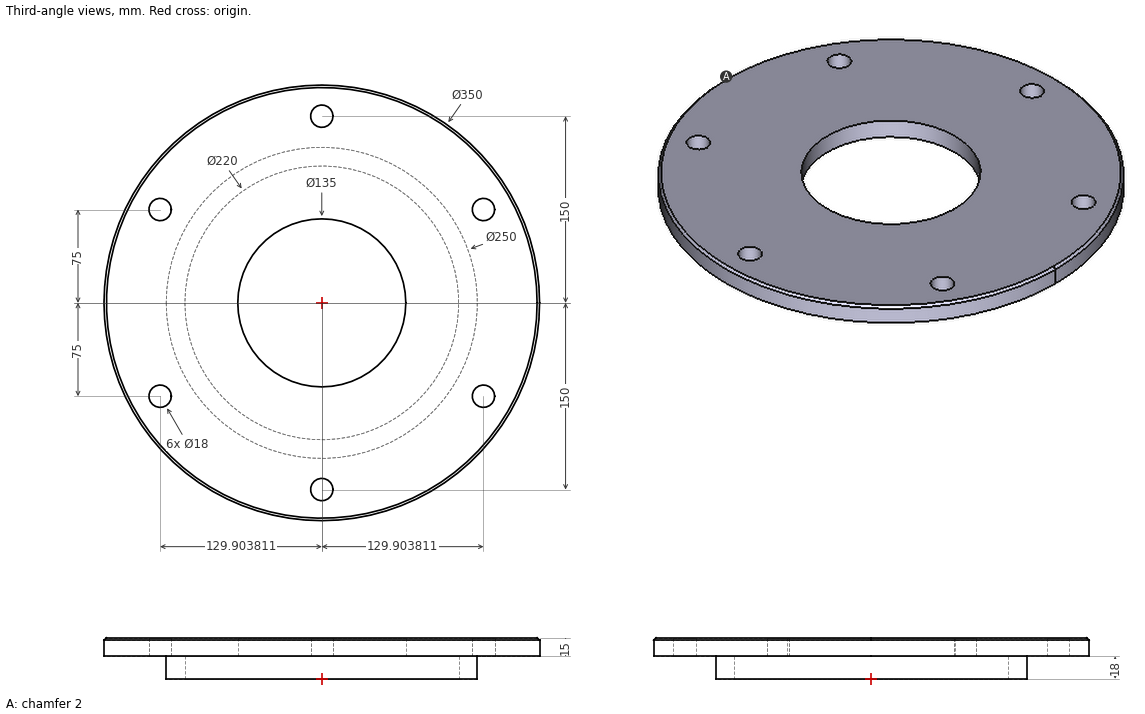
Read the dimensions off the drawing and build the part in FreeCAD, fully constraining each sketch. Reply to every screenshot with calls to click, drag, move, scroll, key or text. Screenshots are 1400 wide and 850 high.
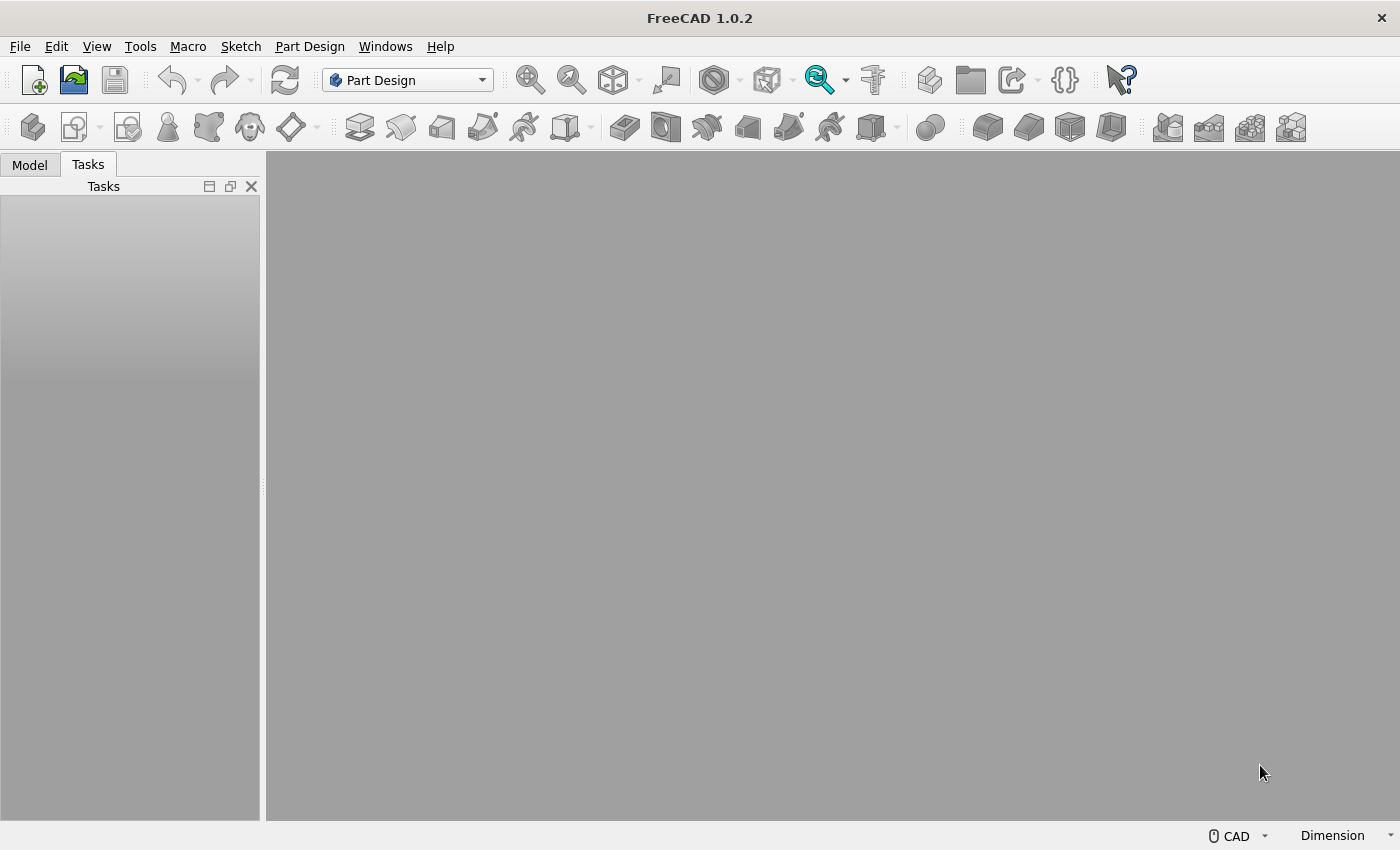
click(33, 80)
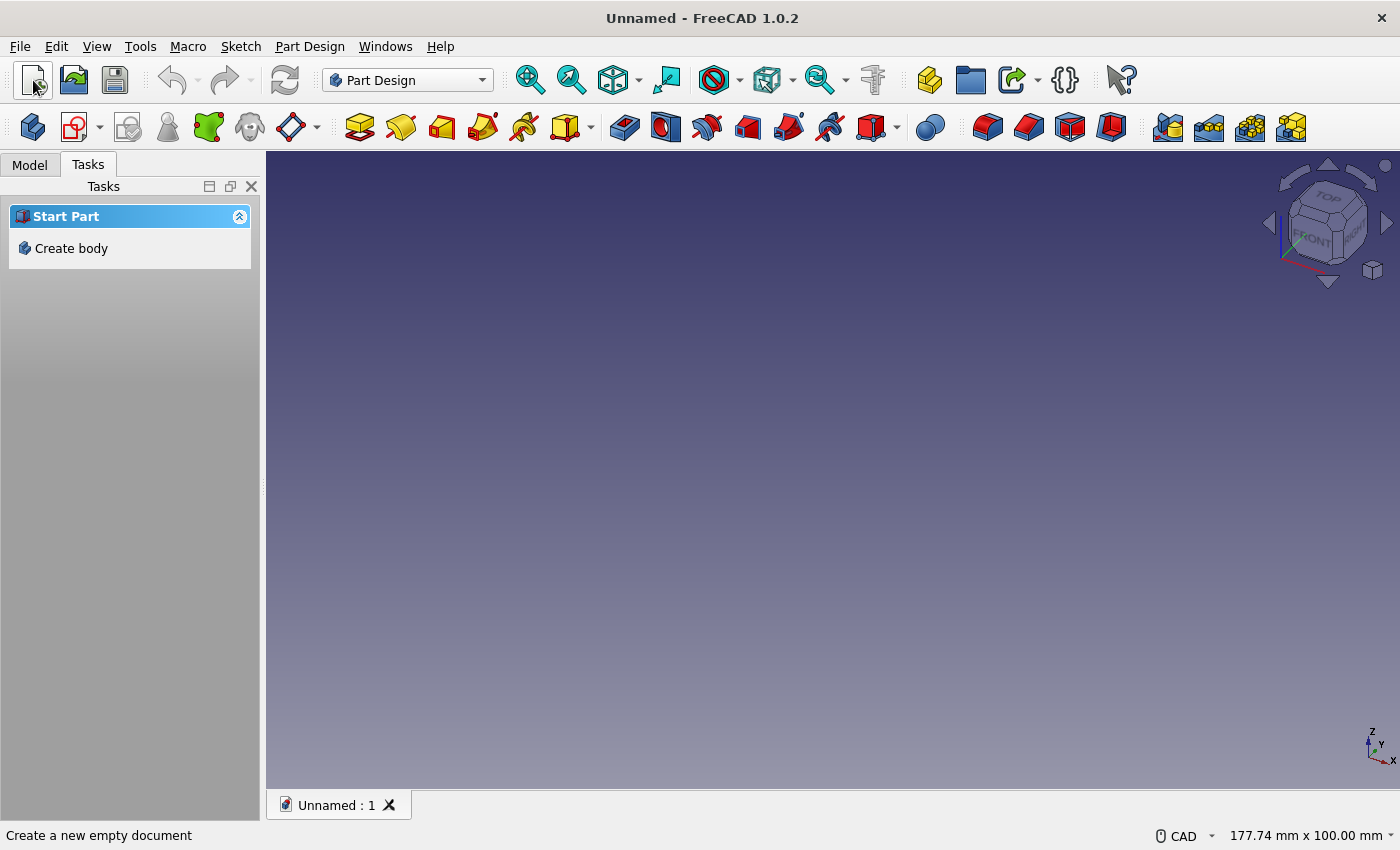
click(74, 128)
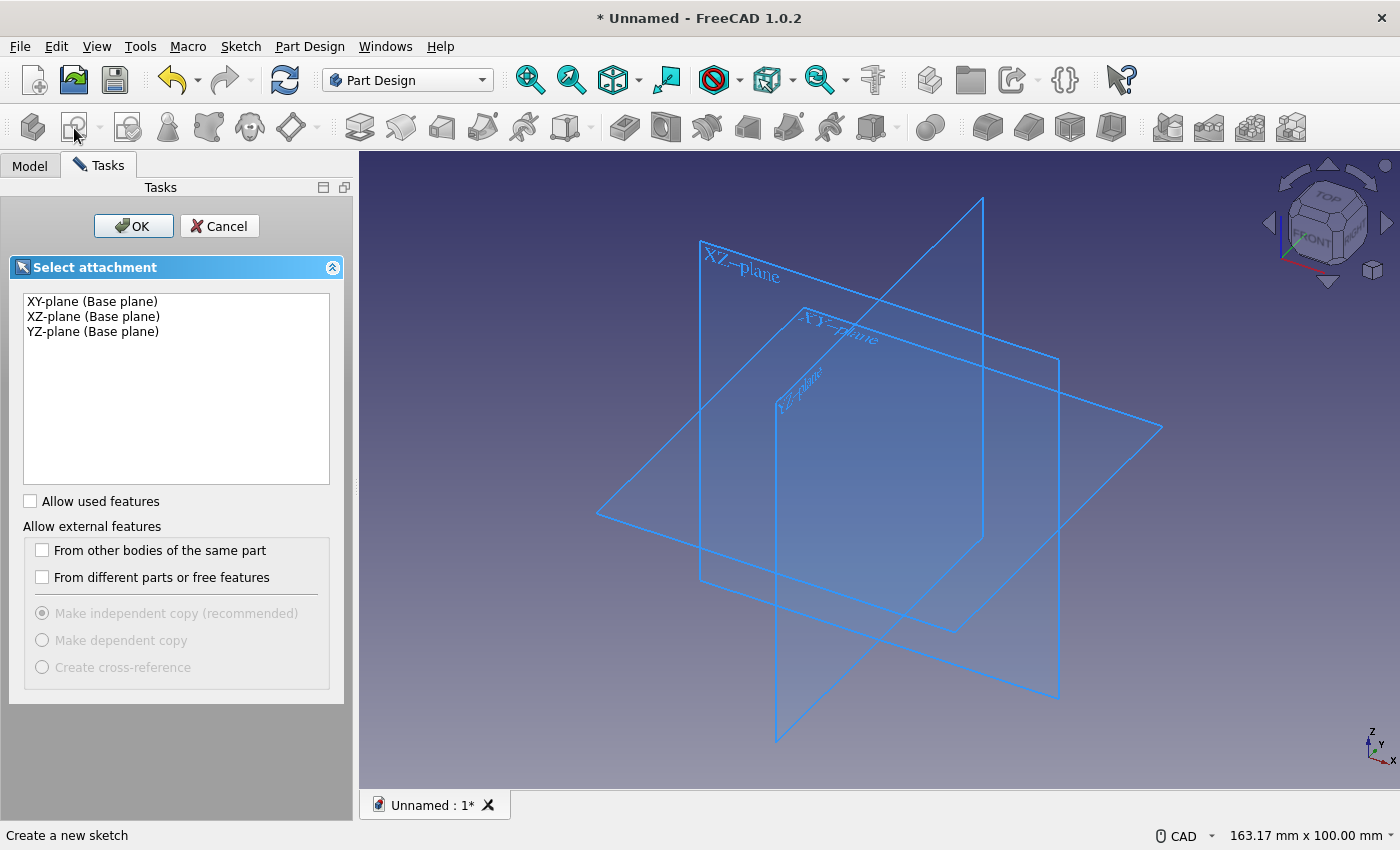
click(84, 302)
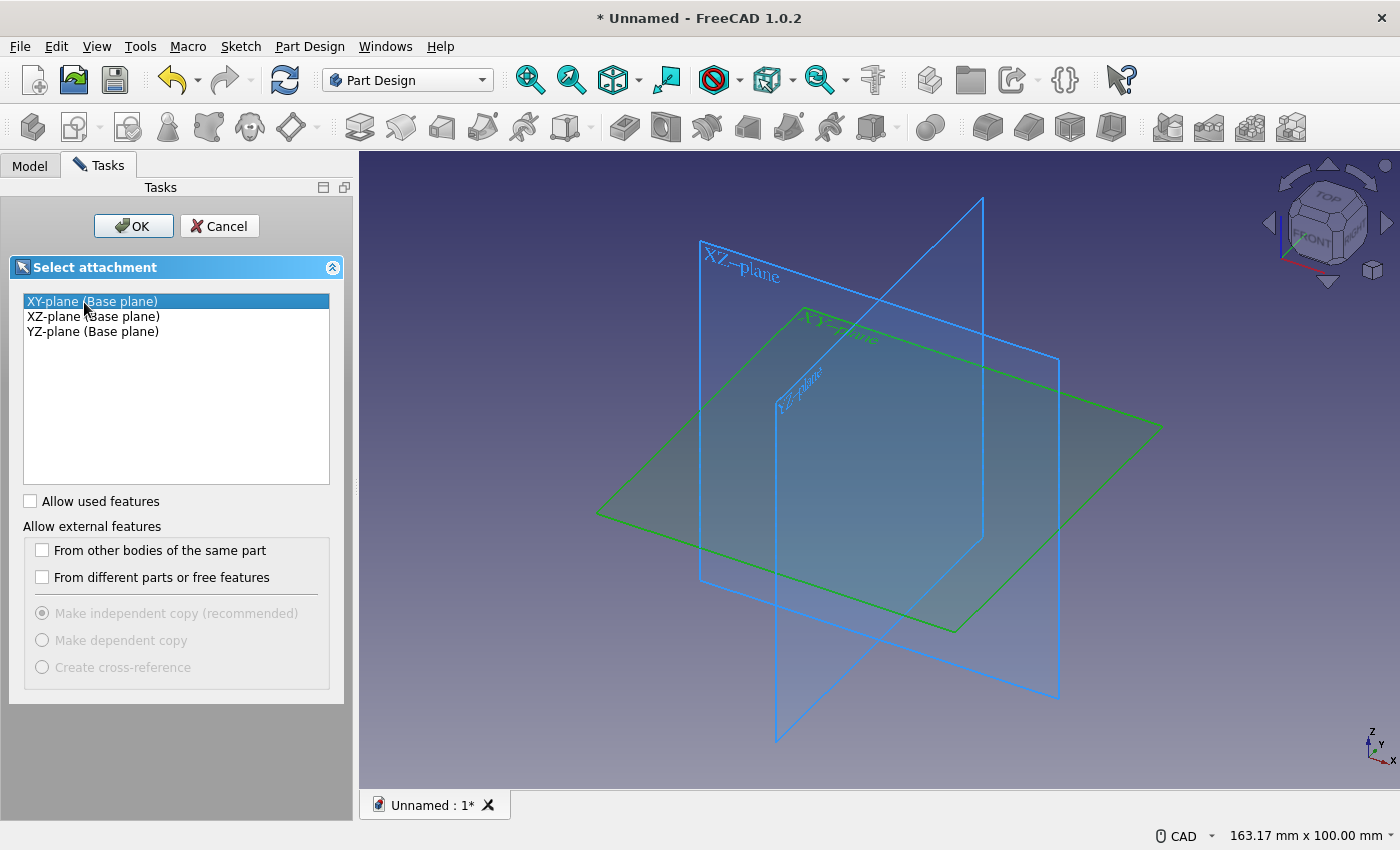
click(134, 226)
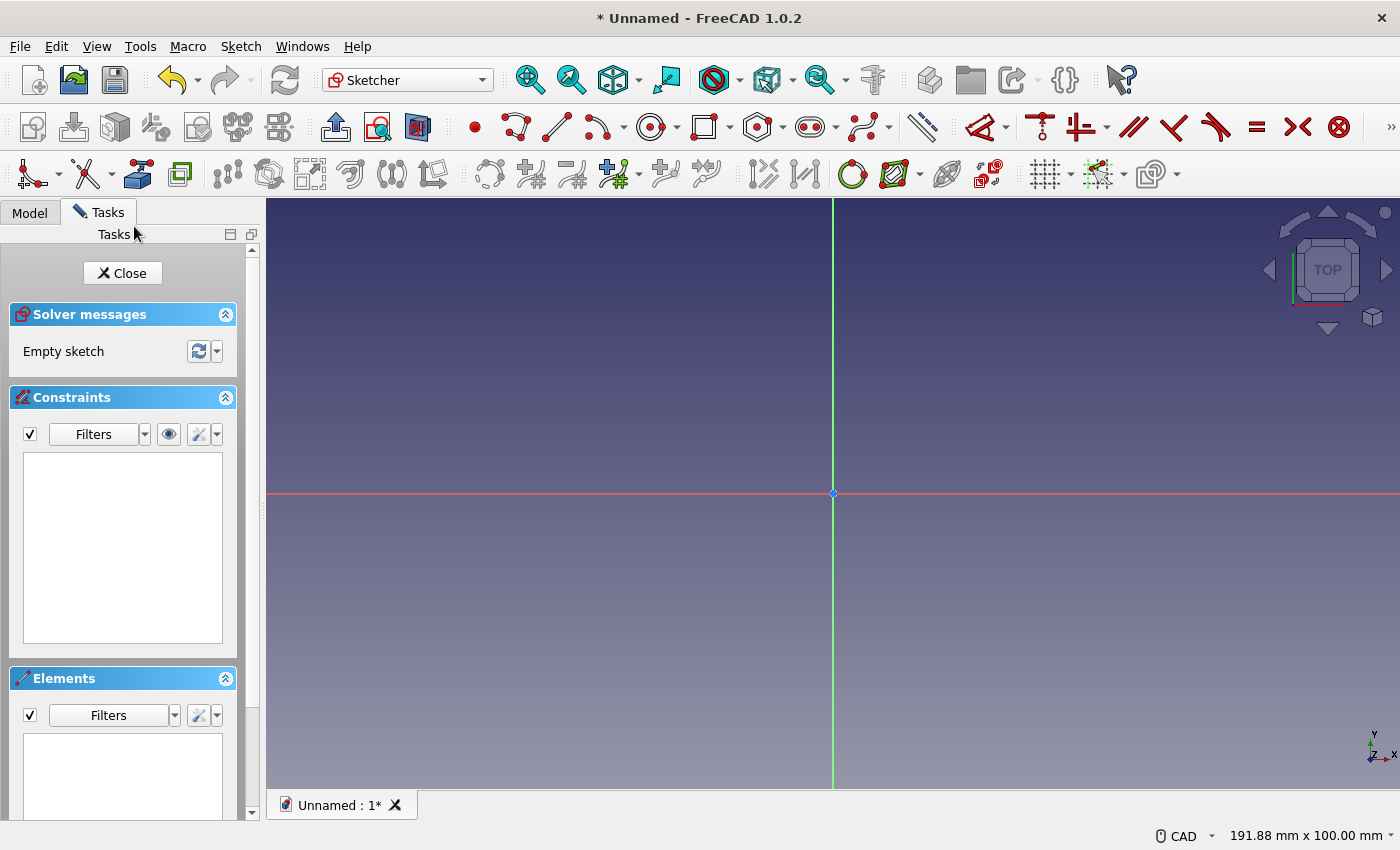
scroll(742, 494, down, 7)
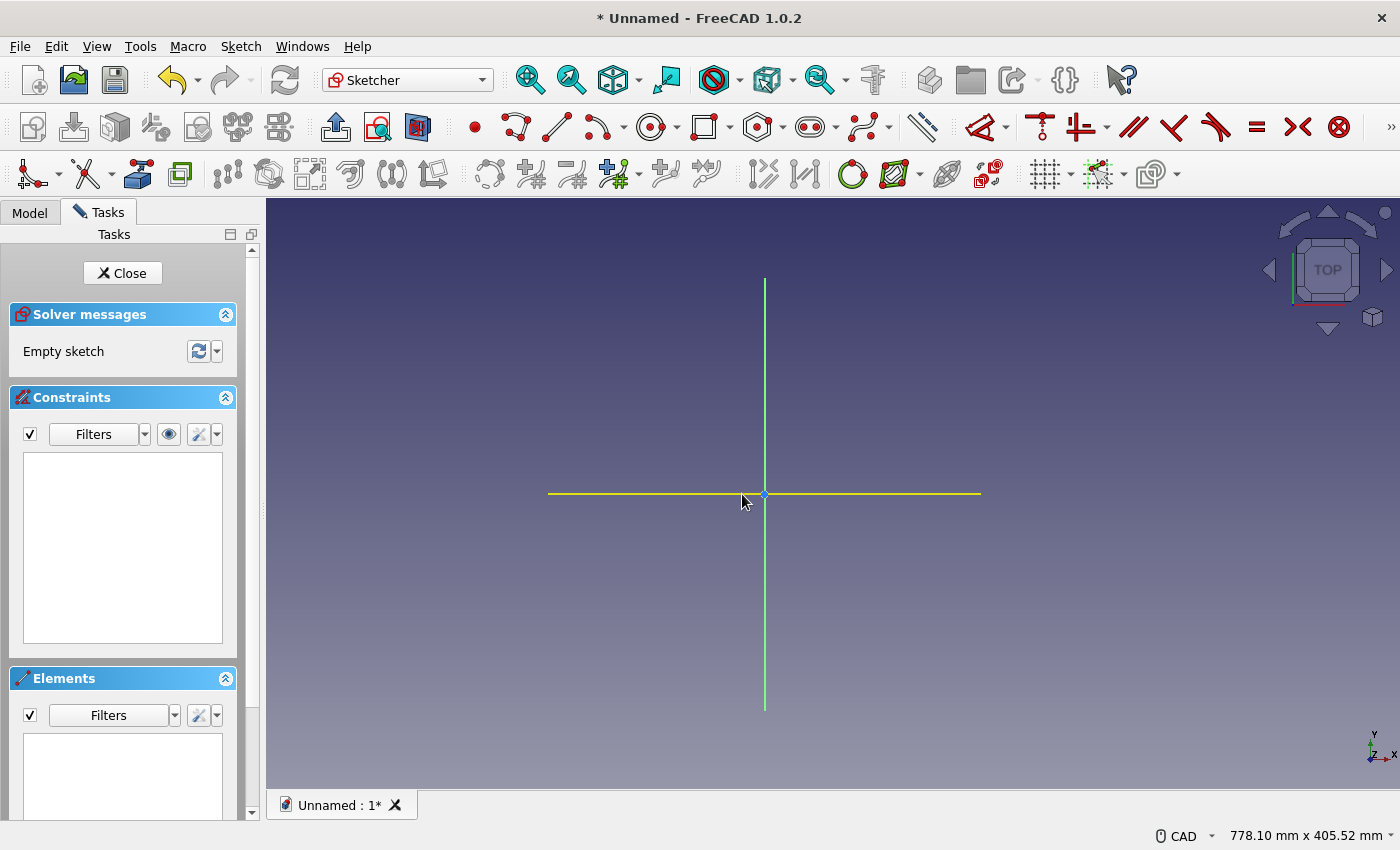
click(650, 128)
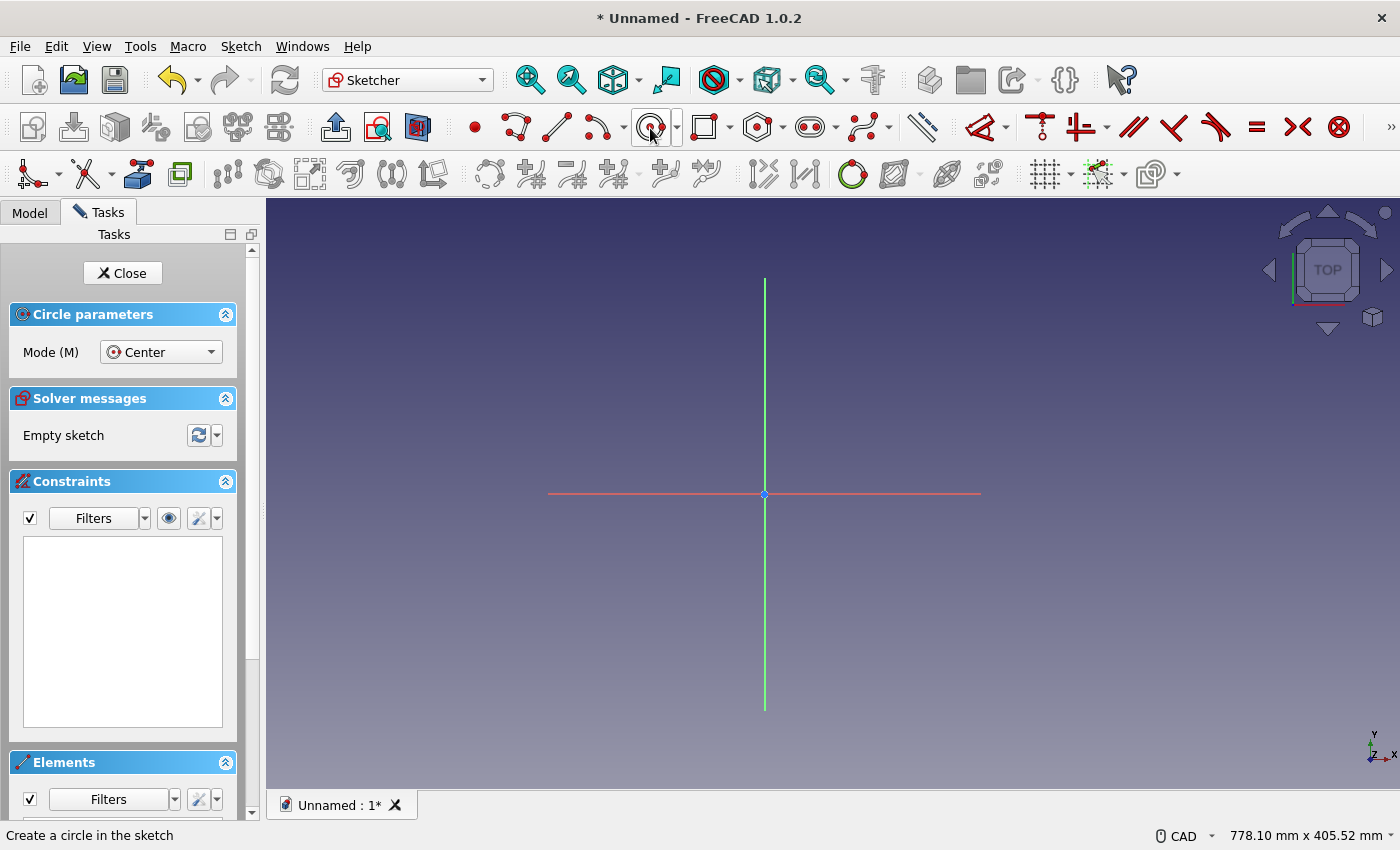
click(765, 494)
click(894, 365)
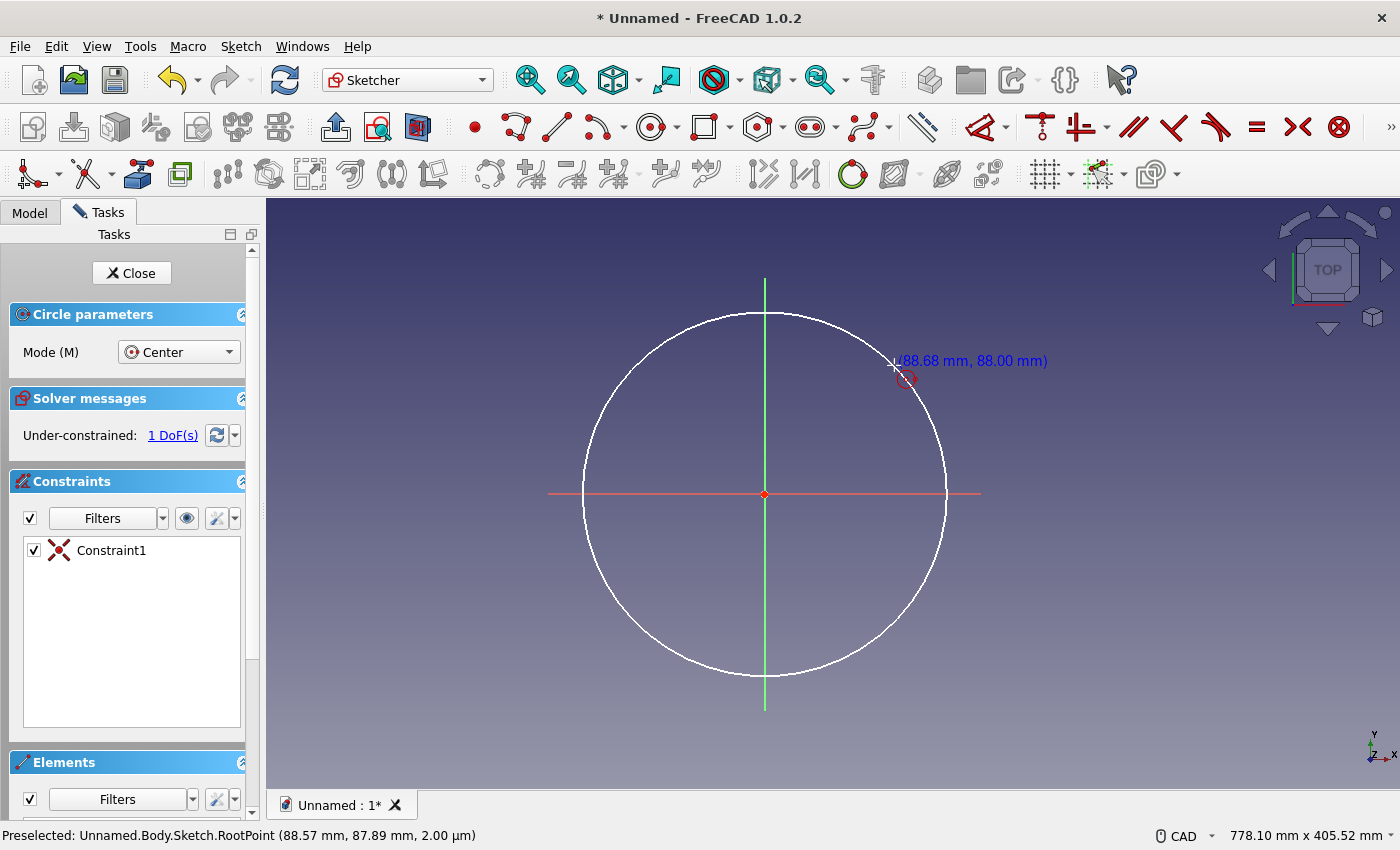
click(765, 494)
click(878, 381)
key(Escape)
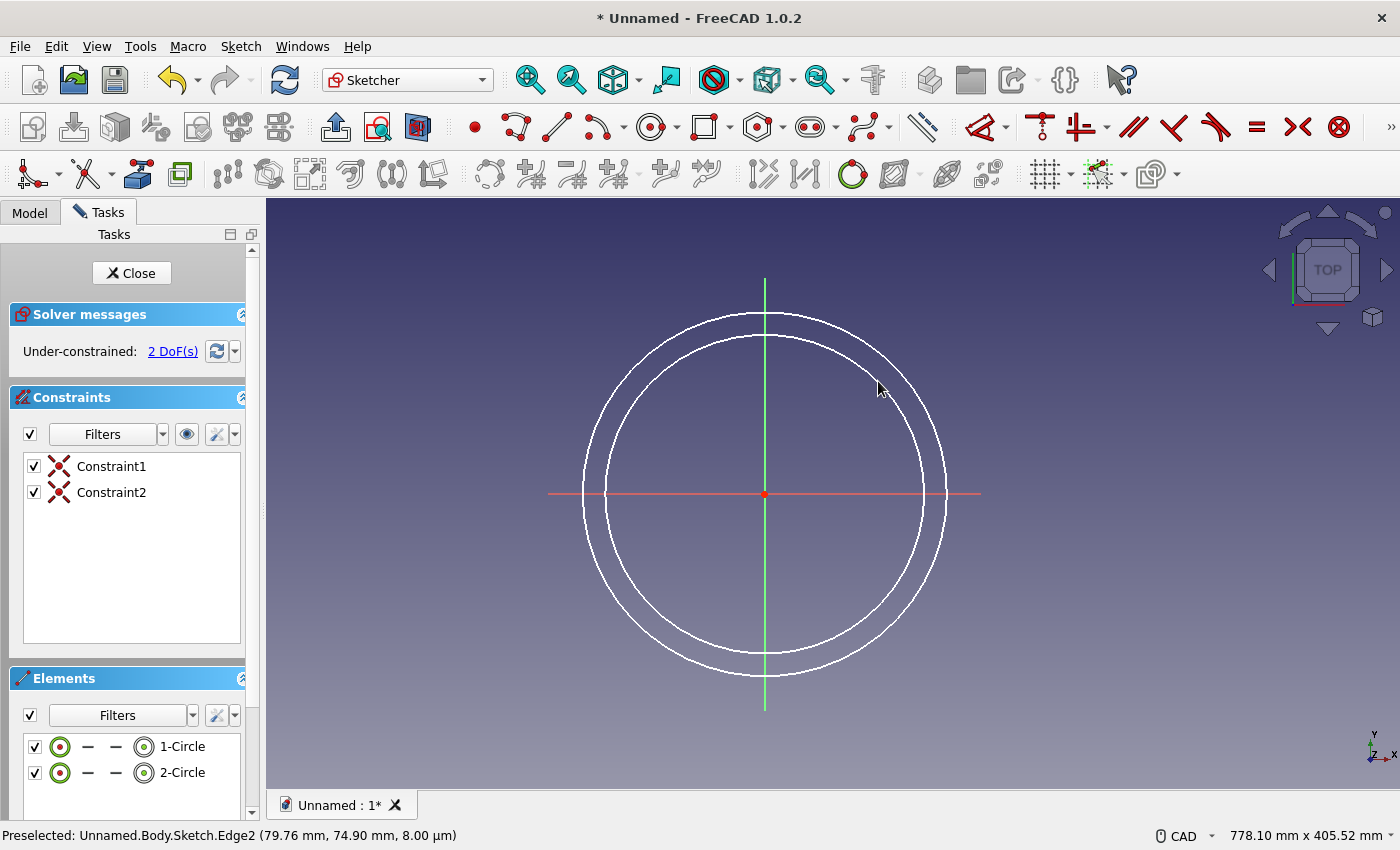
click(893, 365)